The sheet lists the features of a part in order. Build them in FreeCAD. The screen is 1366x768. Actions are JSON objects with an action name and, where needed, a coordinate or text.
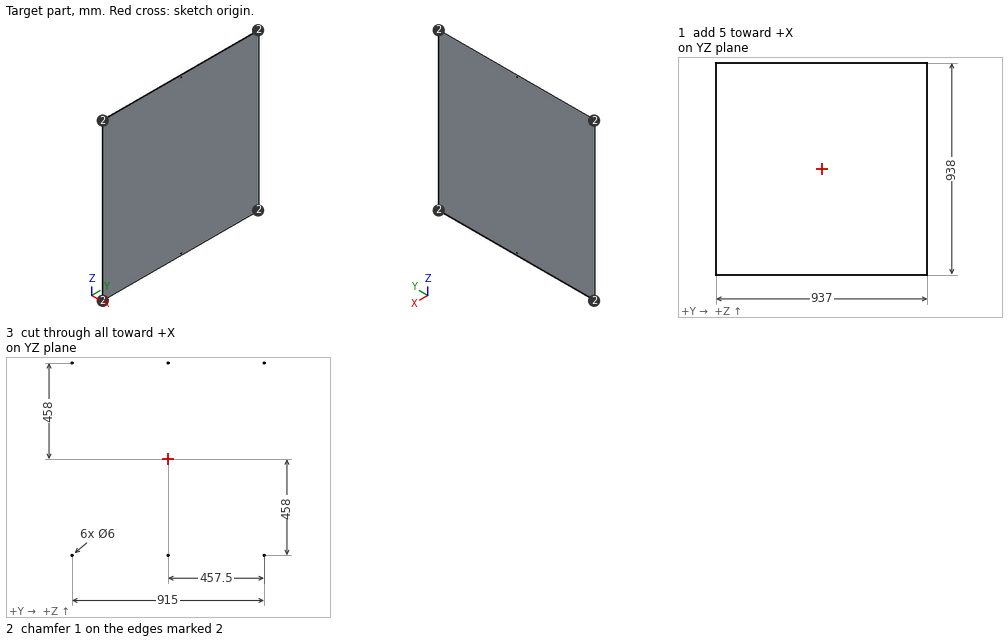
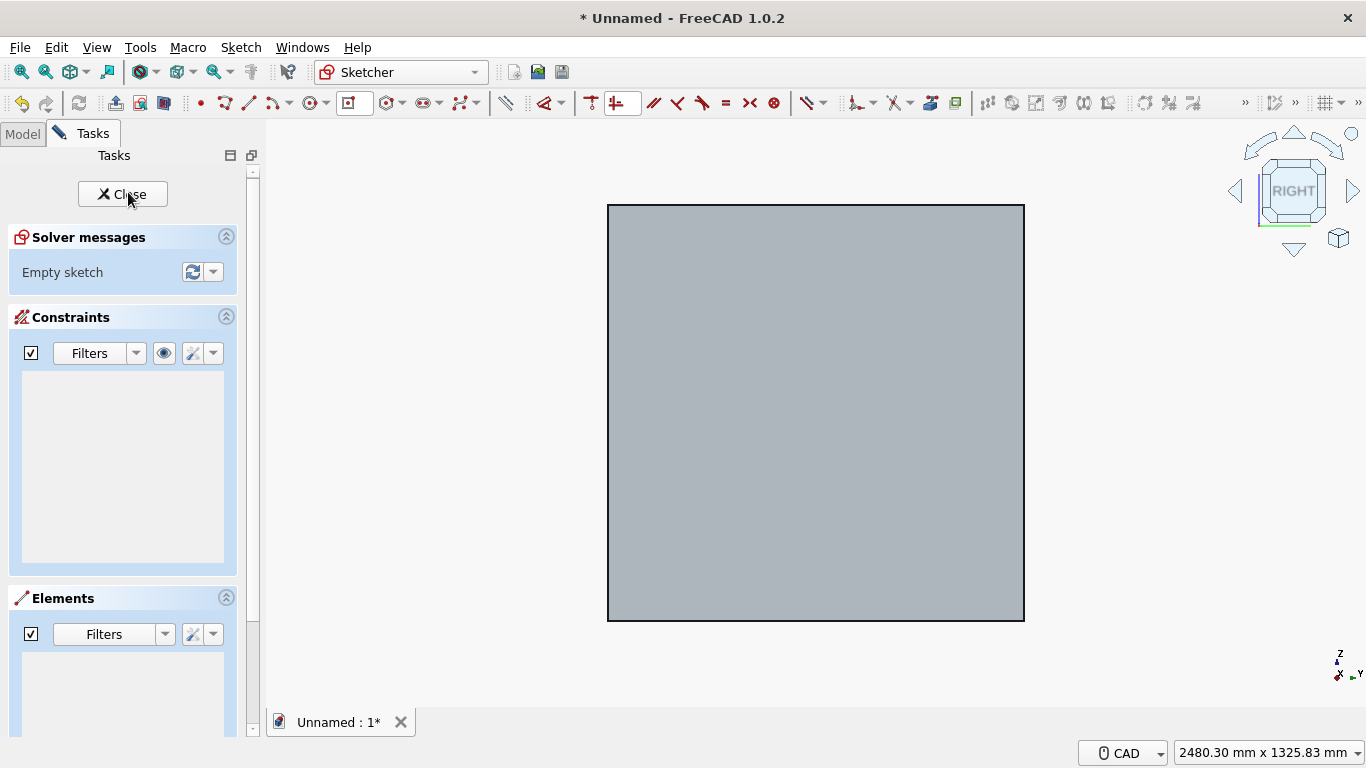
{"action": "left_click", "coordinate": [164, 104]}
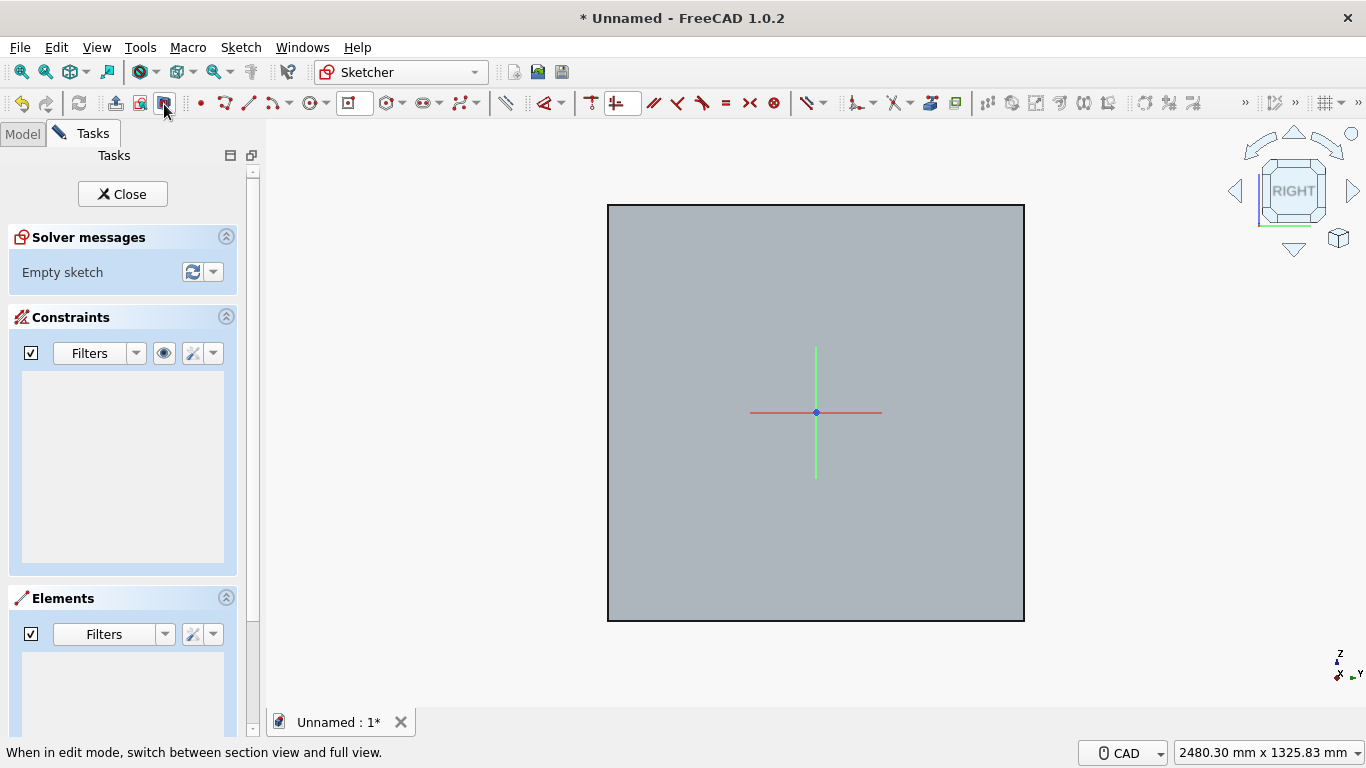
{"action": "left_click", "coordinate": [310, 104]}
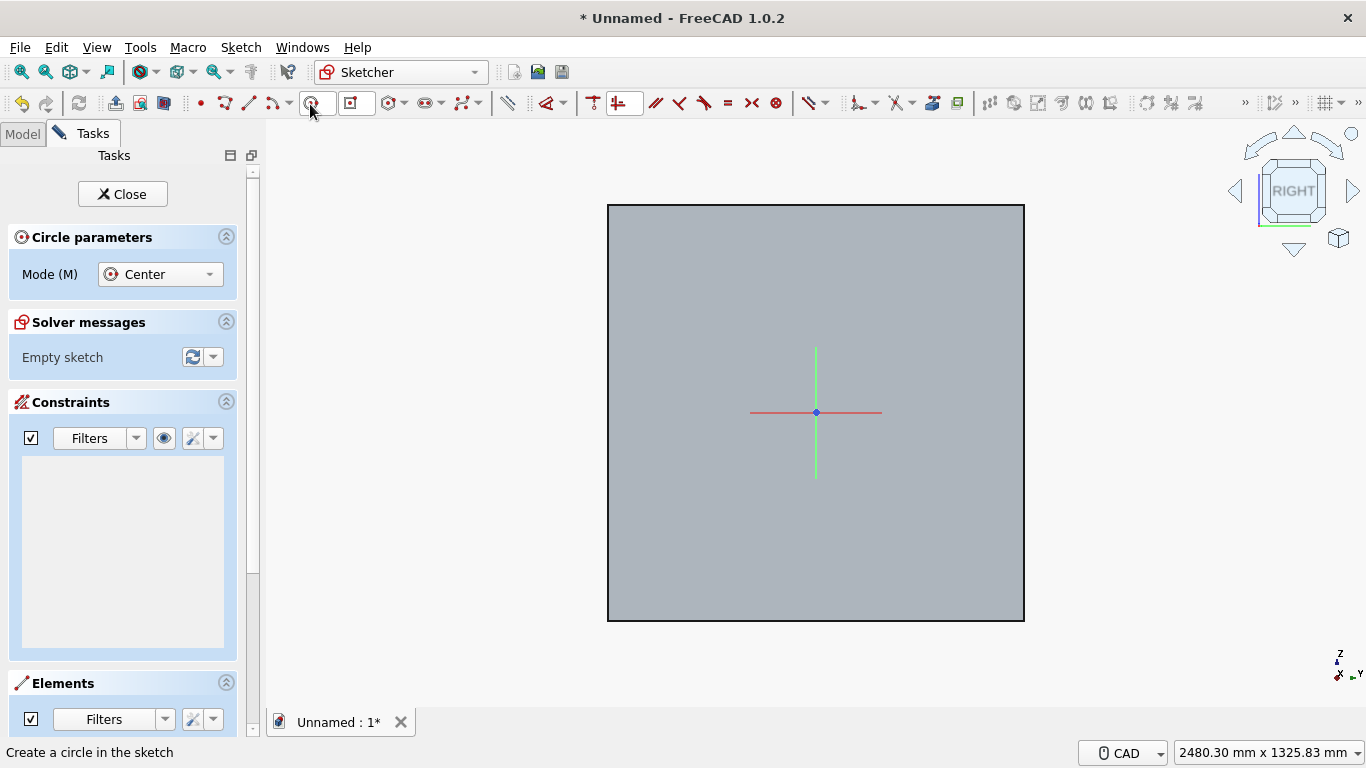
{"action": "scroll", "coordinate": [1019, 616], "scroll_direction": "up", "scroll_amount": 15}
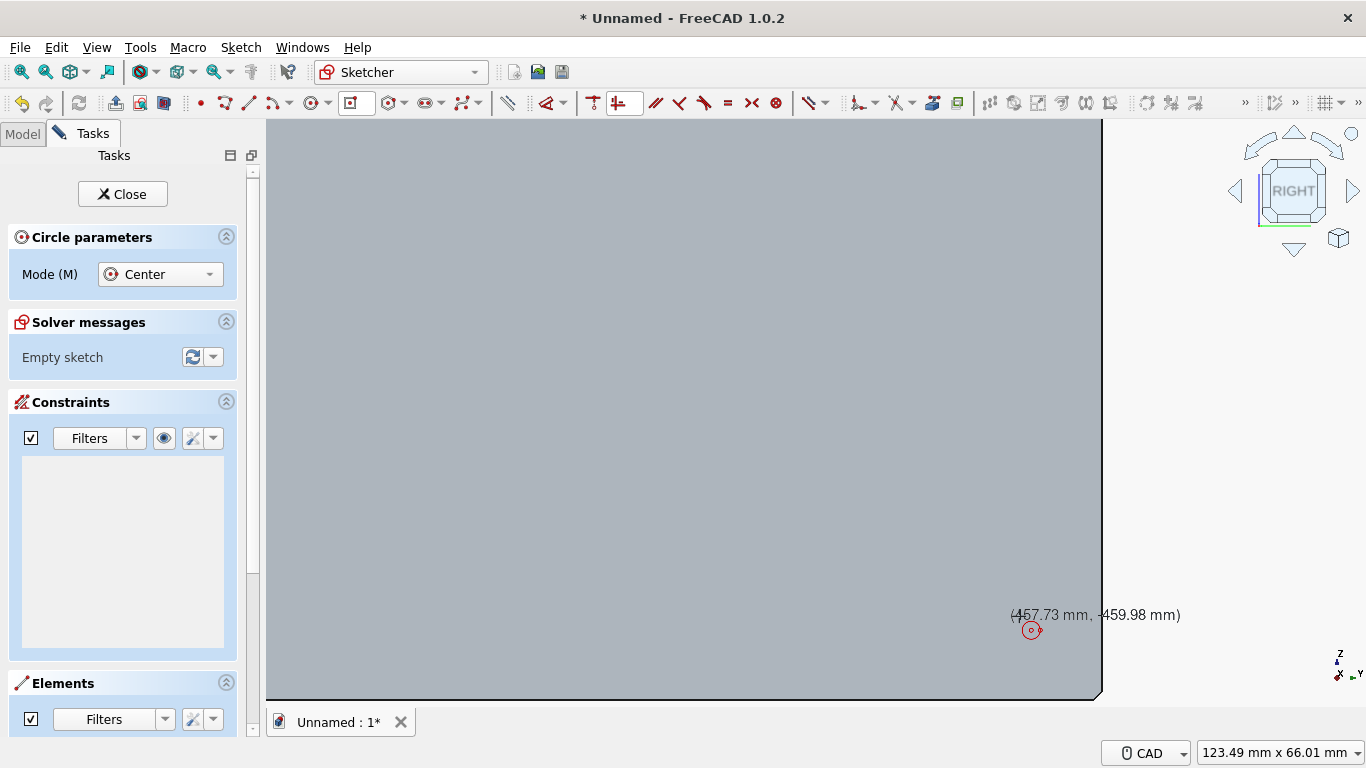
{"action": "scroll", "coordinate": [948, 617], "scroll_direction": "down", "scroll_amount": 15}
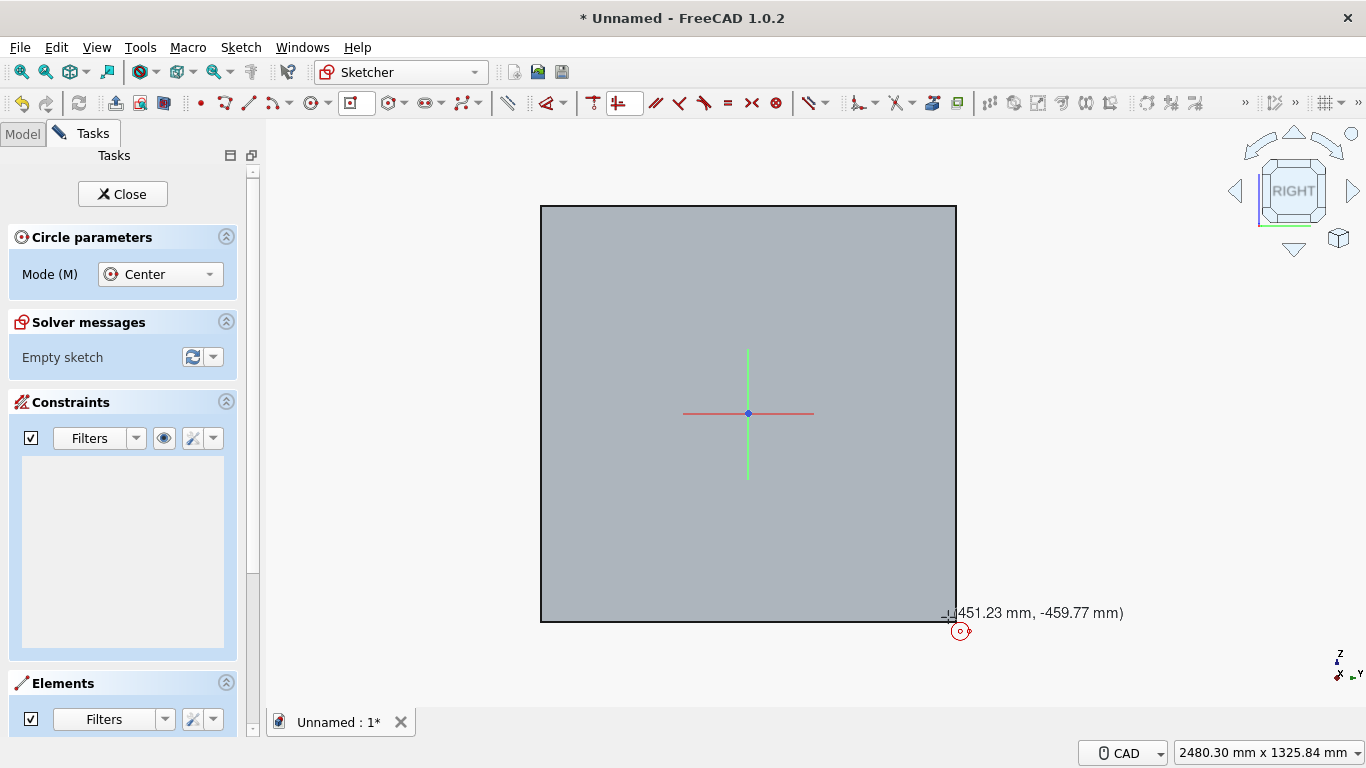
{"action": "left_click", "coordinate": [951, 617]}
{"action": "mouse_move", "coordinate": [952, 616]}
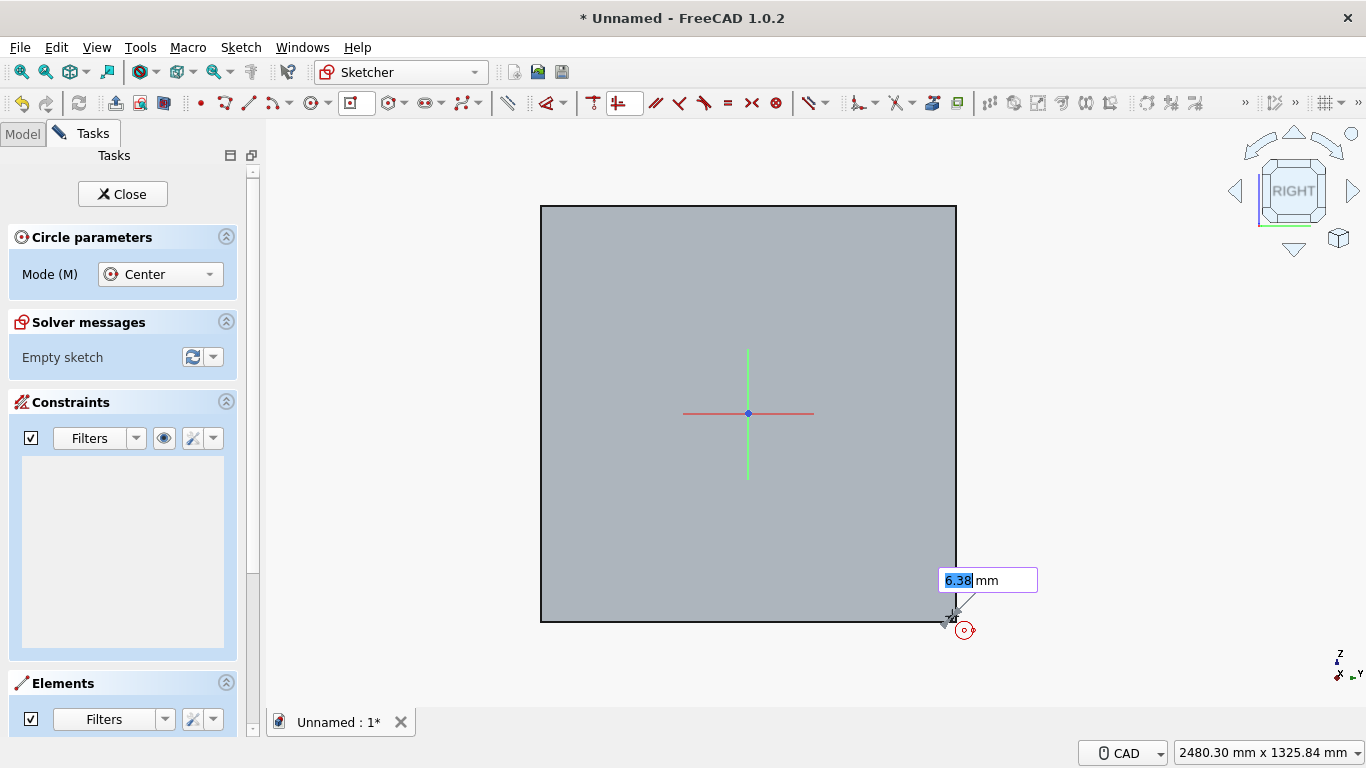
{"action": "type", "text": "6"}
{"action": "key", "text": "Return"}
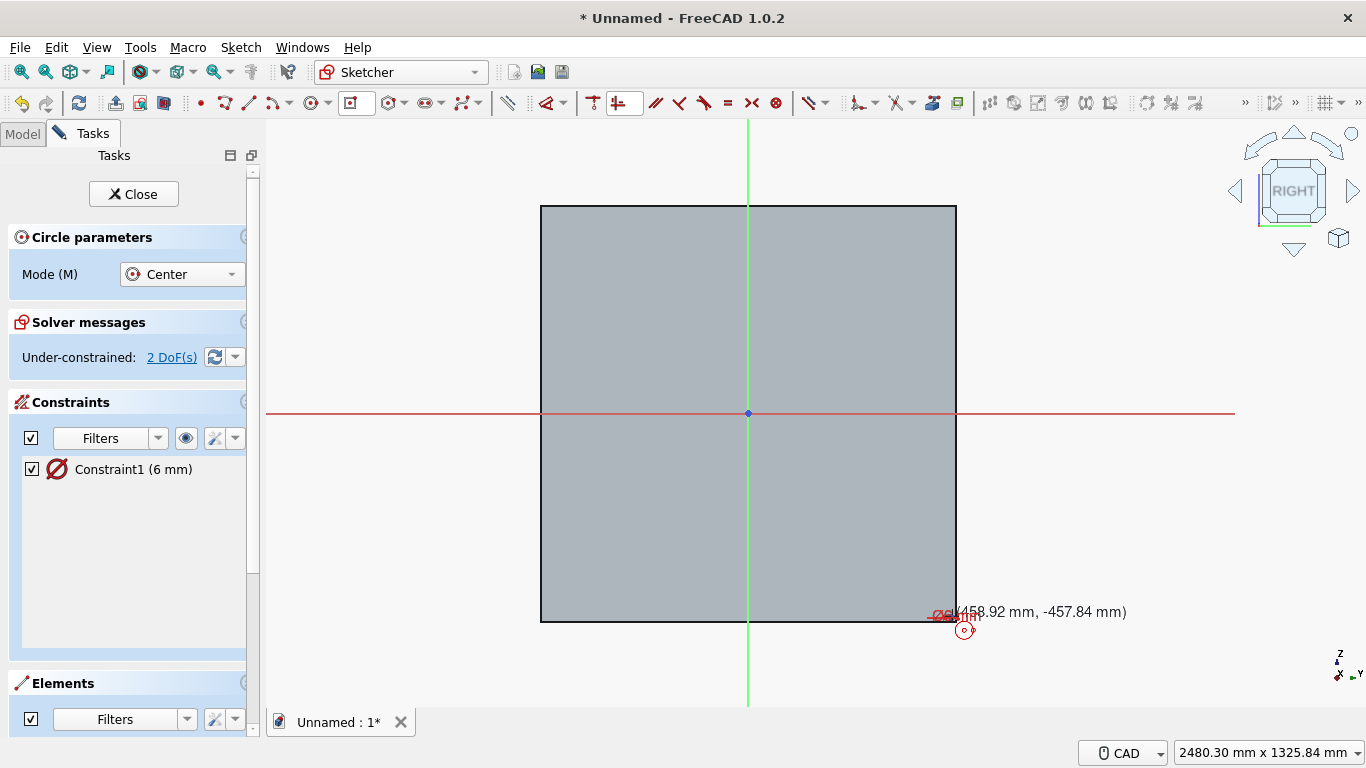
{"action": "scroll", "coordinate": [546, 617], "scroll_direction": "up", "scroll_amount": 15}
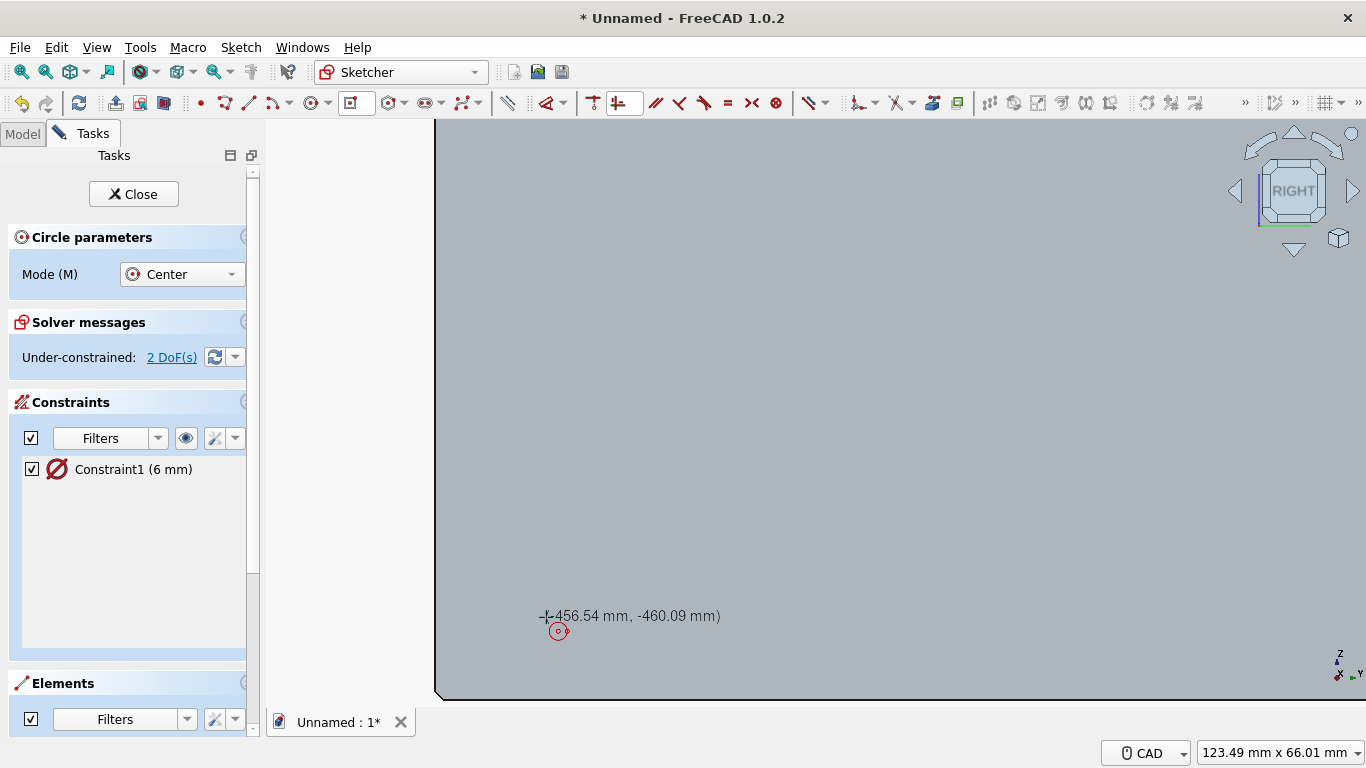
{"action": "scroll", "coordinate": [545, 617], "scroll_direction": "down", "scroll_amount": 15}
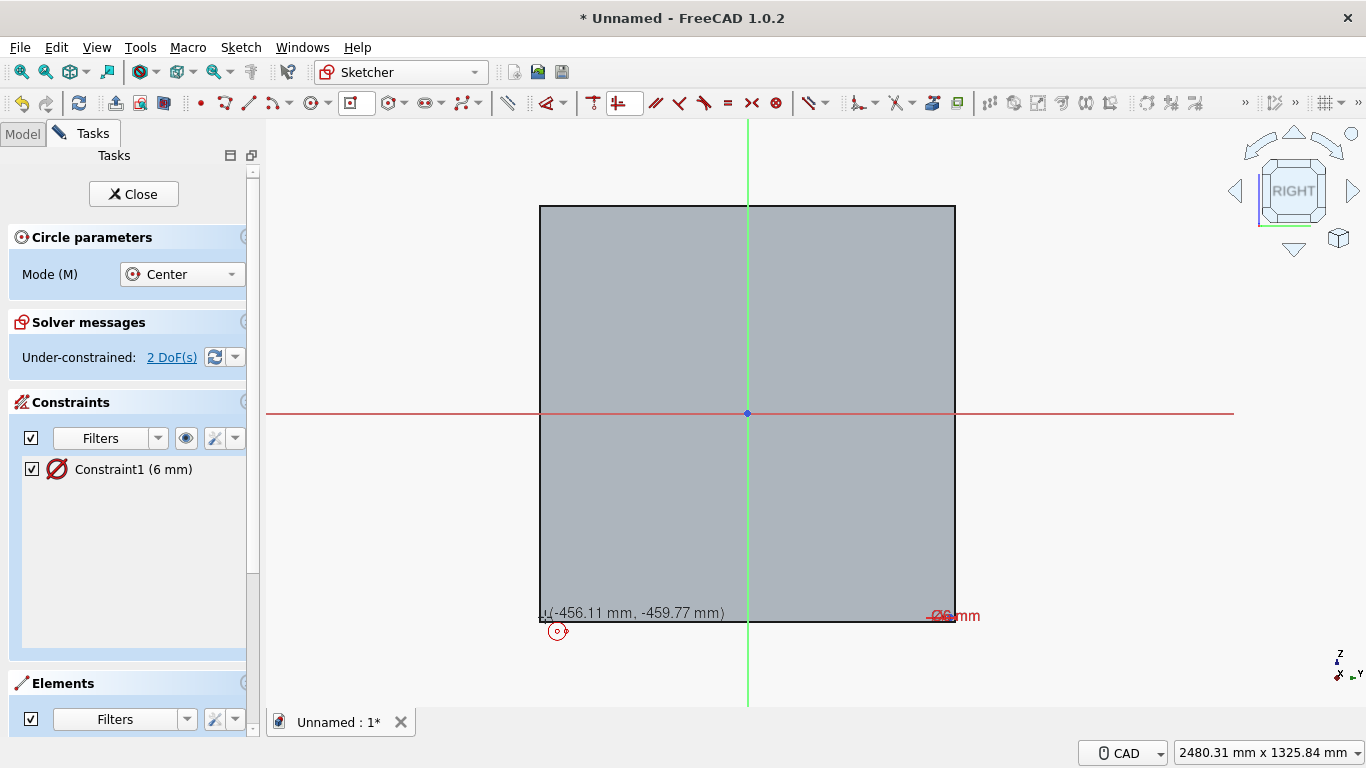
{"action": "left_click", "coordinate": [545, 617]}
{"action": "mouse_move", "coordinate": [546, 616]}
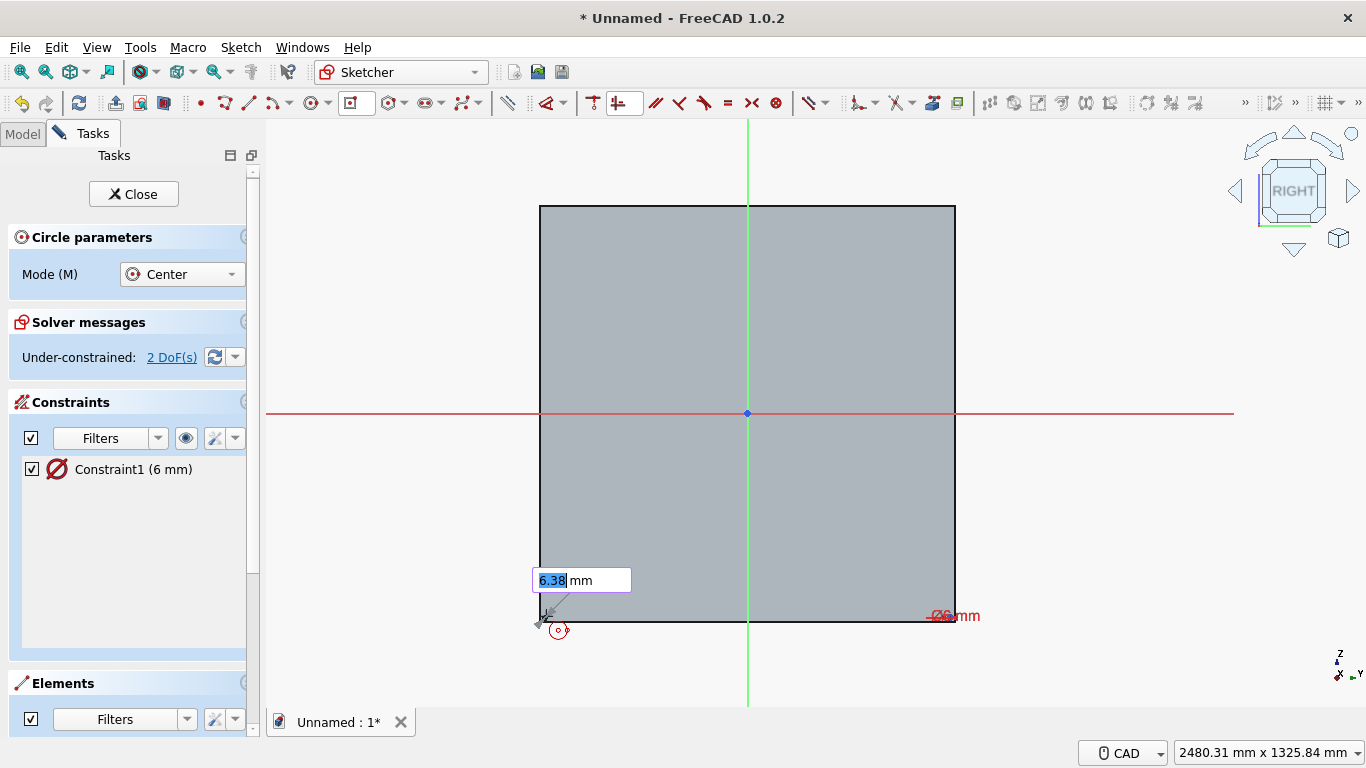
{"action": "type", "text": "6"}
{"action": "key", "text": "Return"}